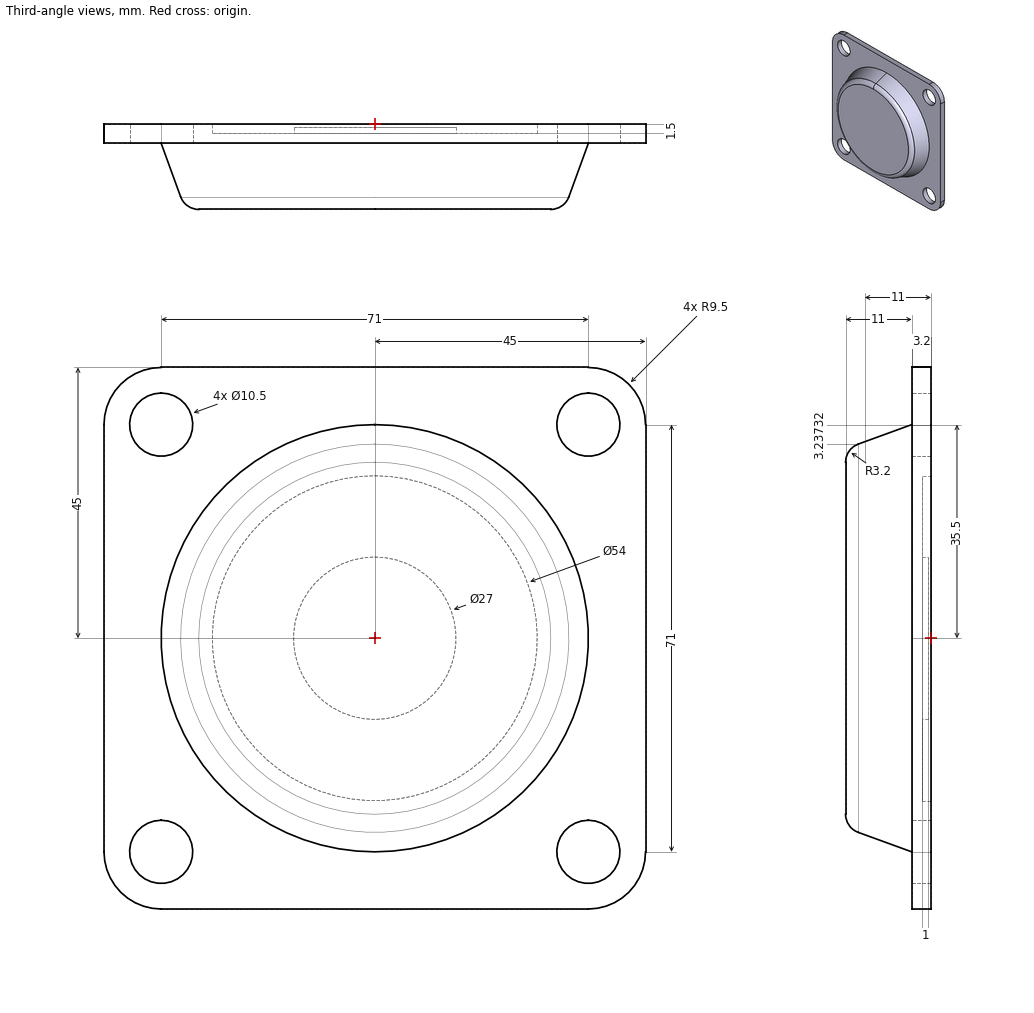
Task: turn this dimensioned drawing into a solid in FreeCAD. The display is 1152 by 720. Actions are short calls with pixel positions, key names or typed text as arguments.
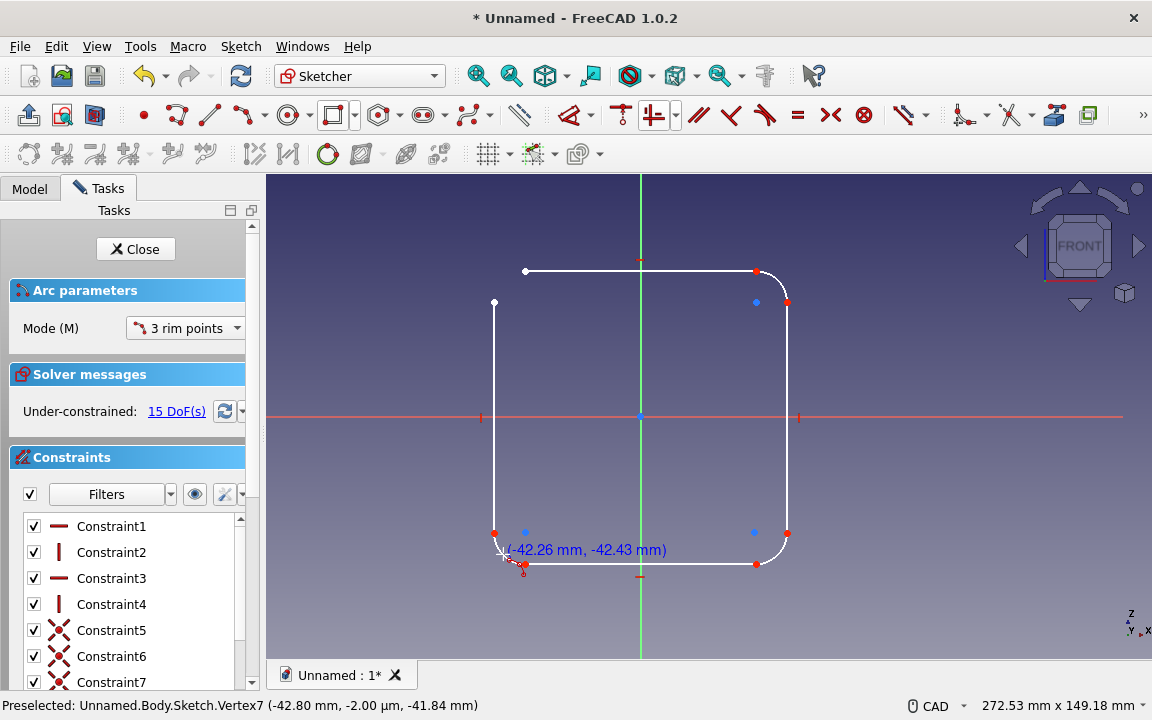
click(494, 302)
click(525, 271)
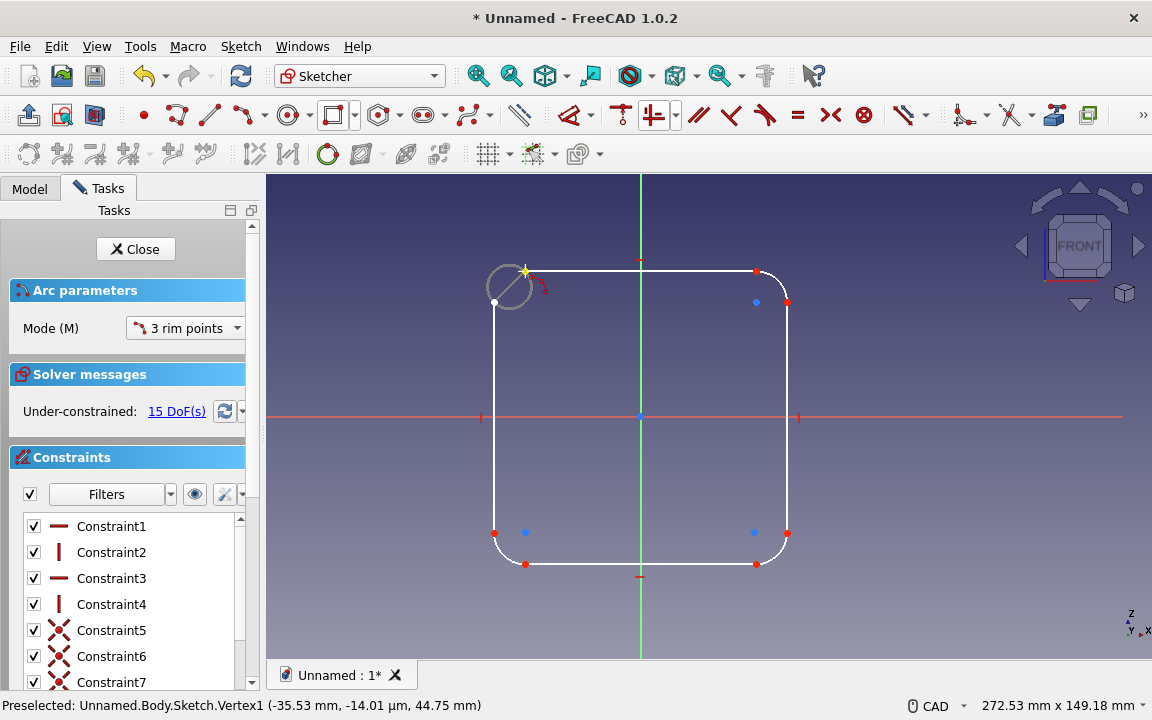
scroll(503, 280, up, 3)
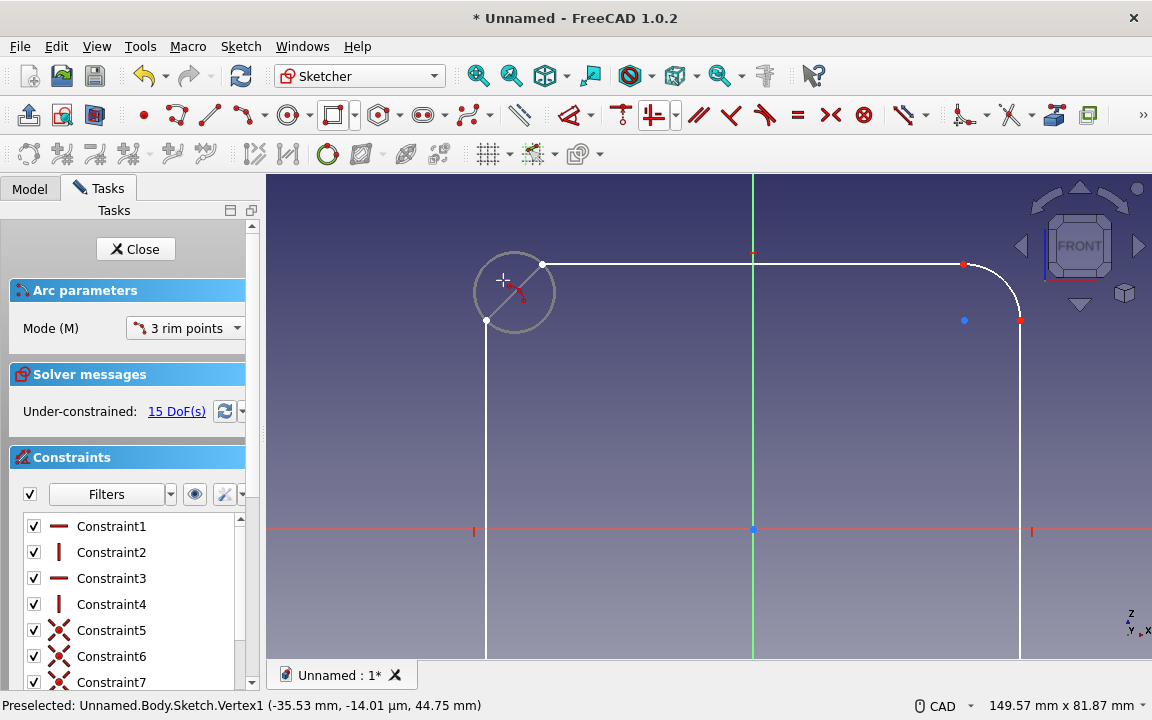
click(503, 279)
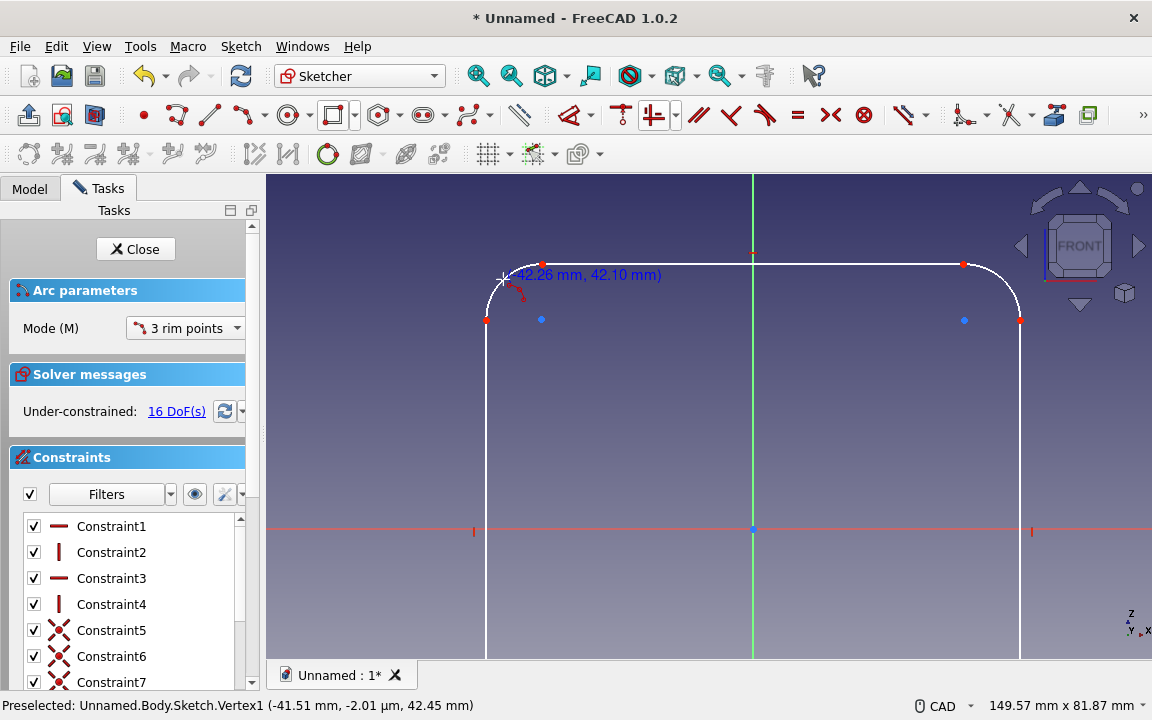
key(g)
key(c)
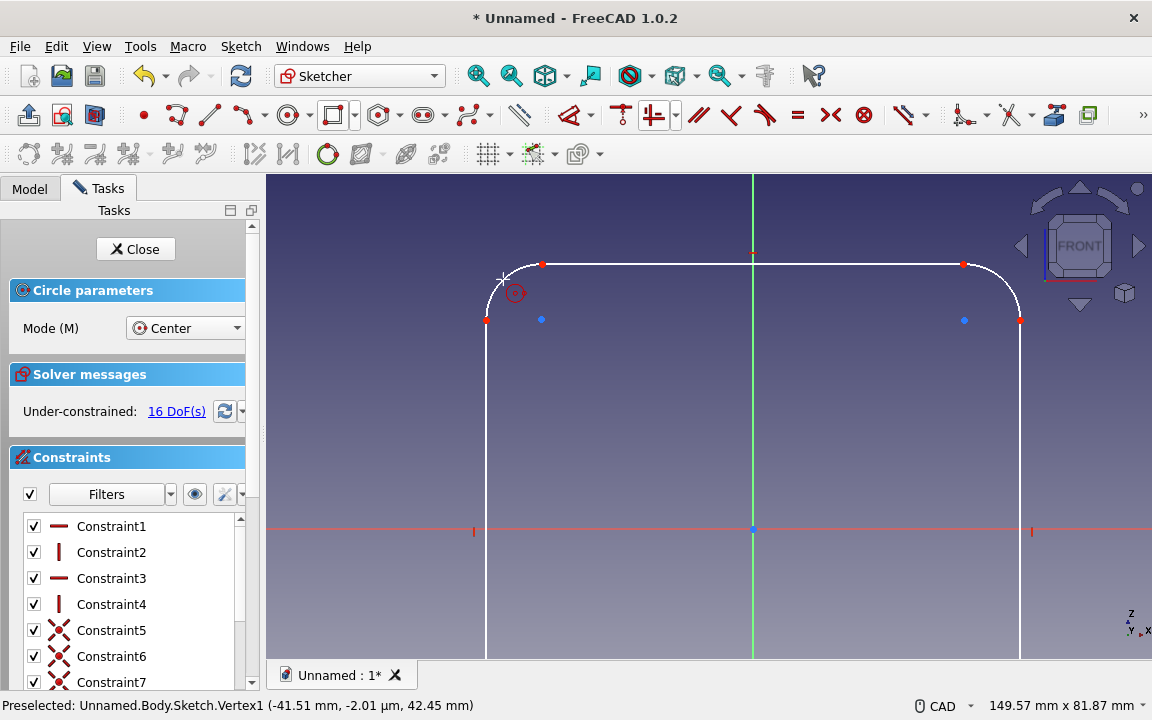
click(543, 319)
move(565, 297)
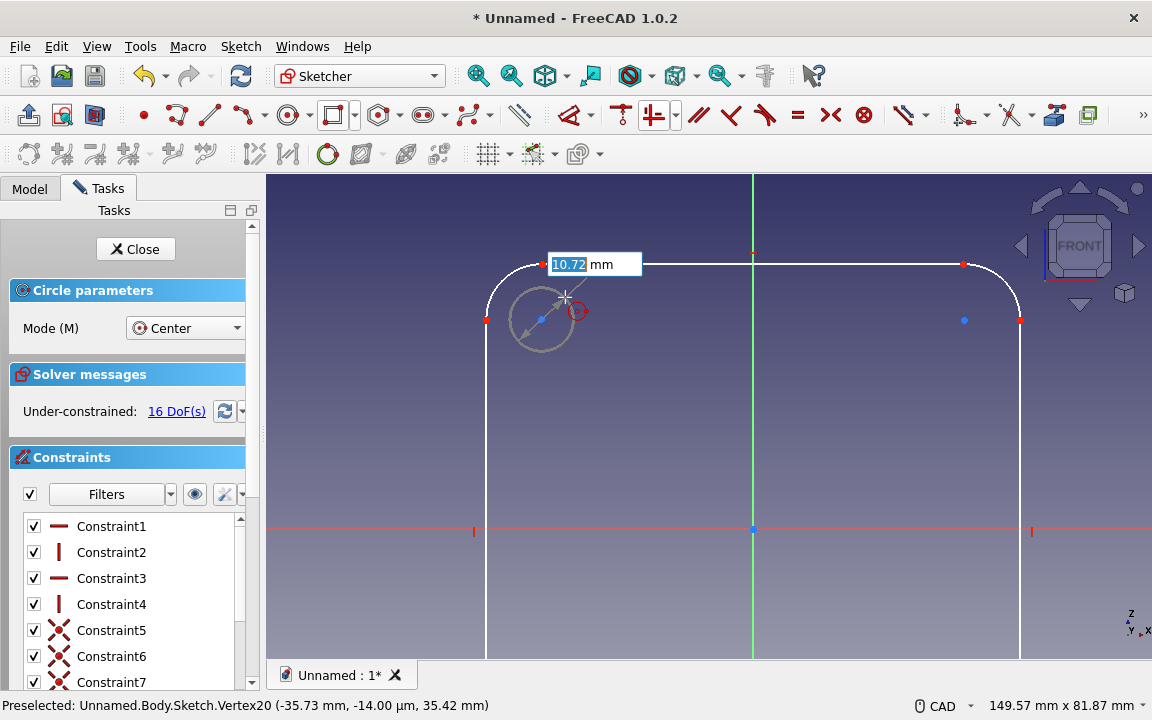
text(10.5)
key(Return)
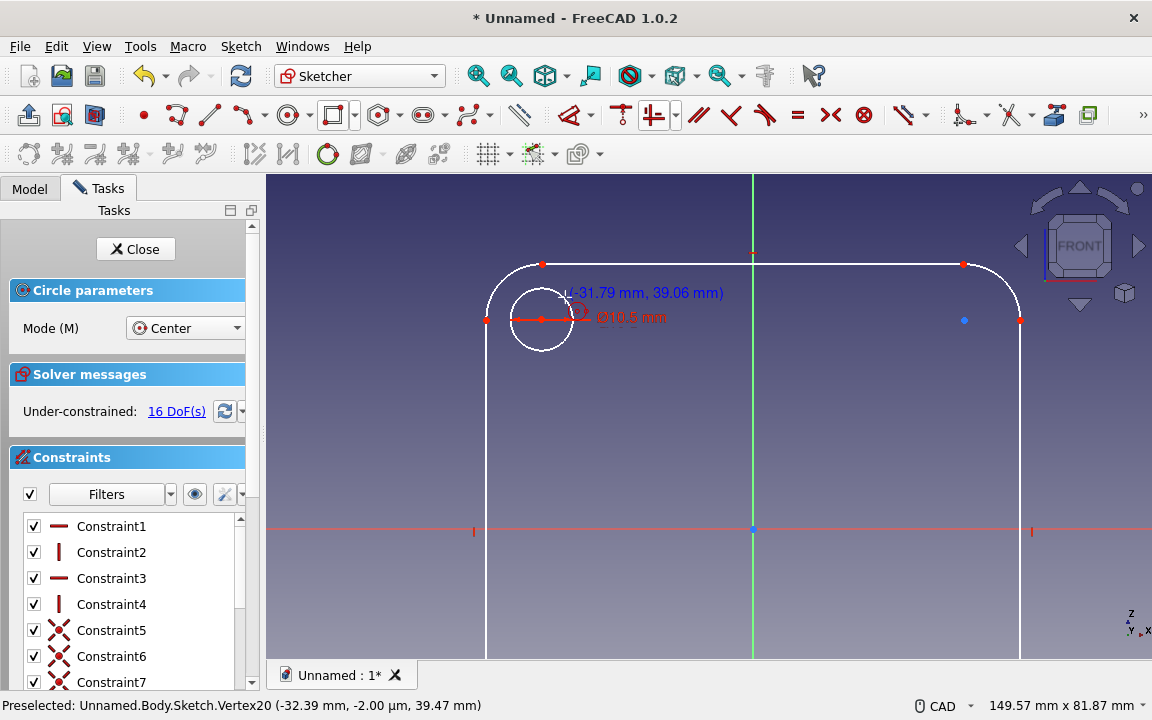
click(964, 319)
move(986, 297)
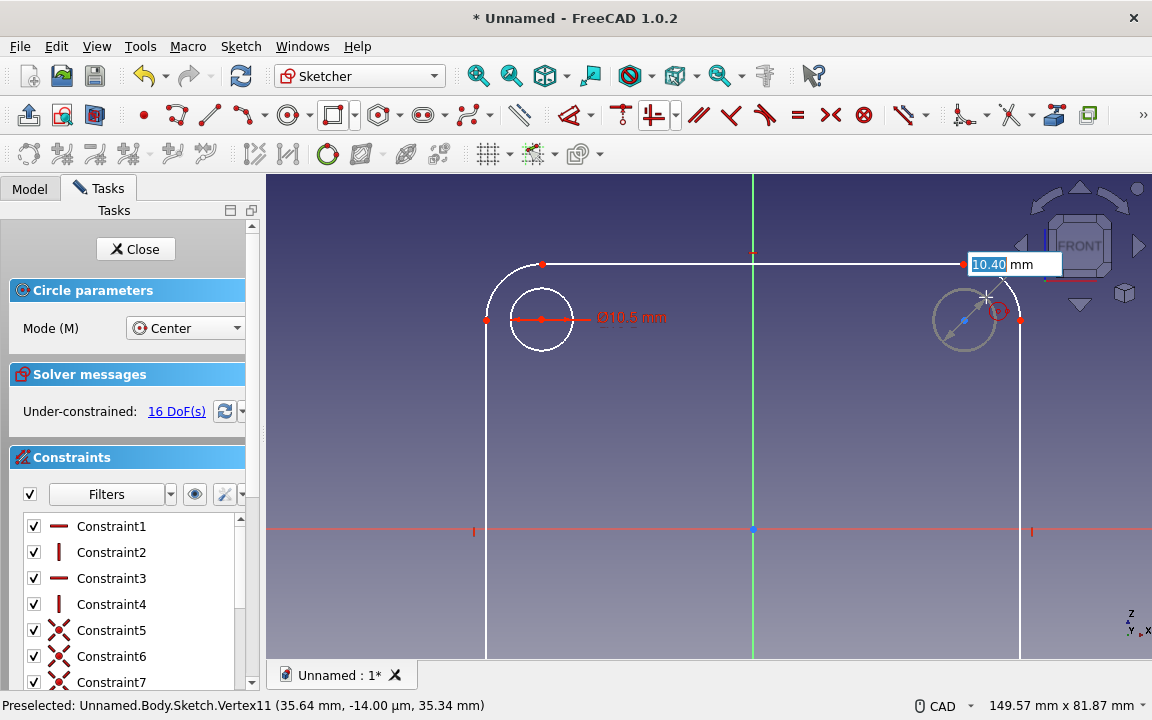
text(10.5)
key(Return)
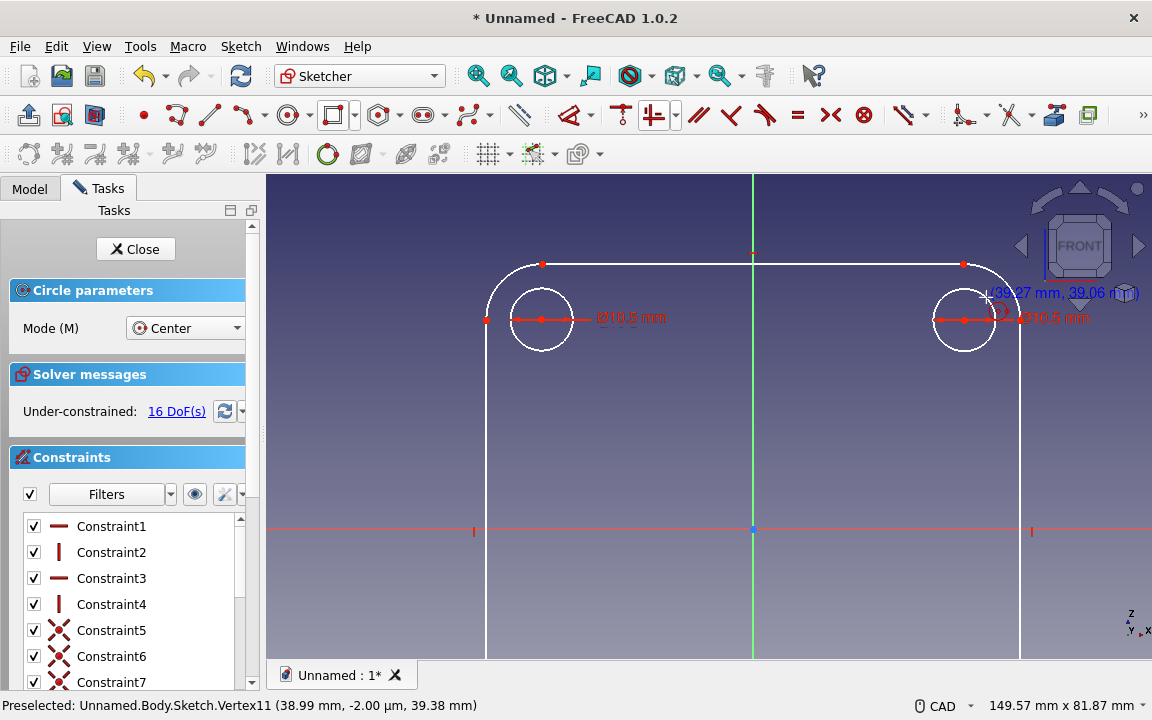
scroll(503, 279, down, 3)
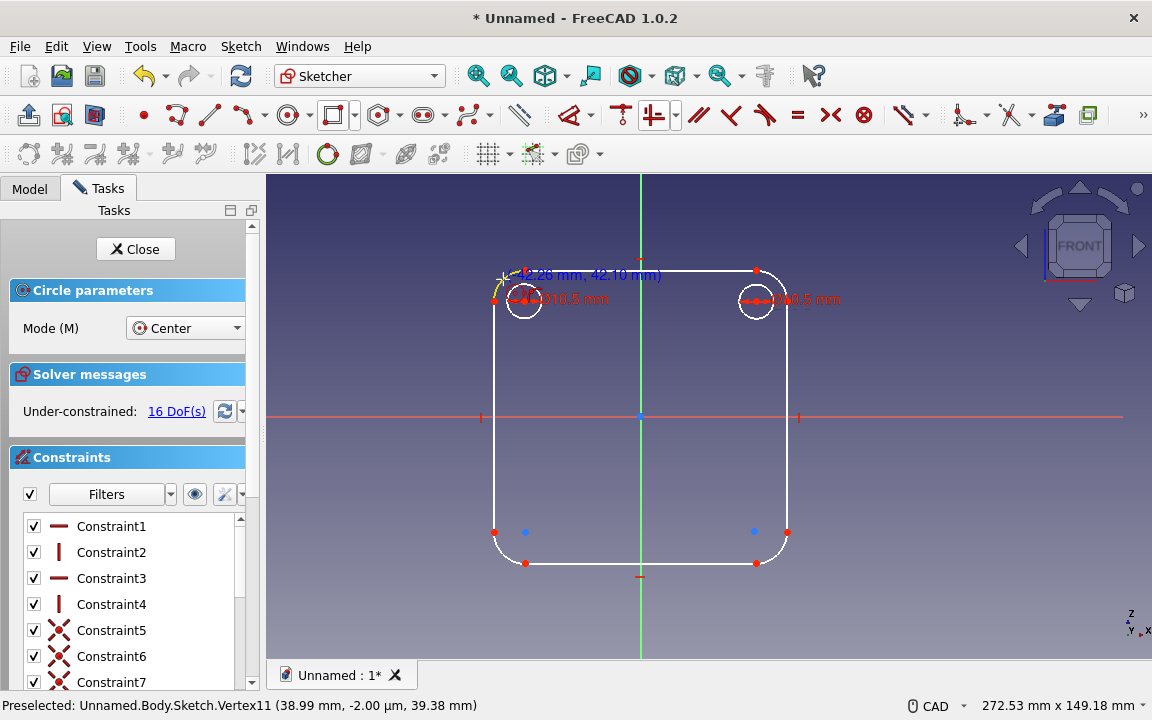
scroll(525, 532, up, 2)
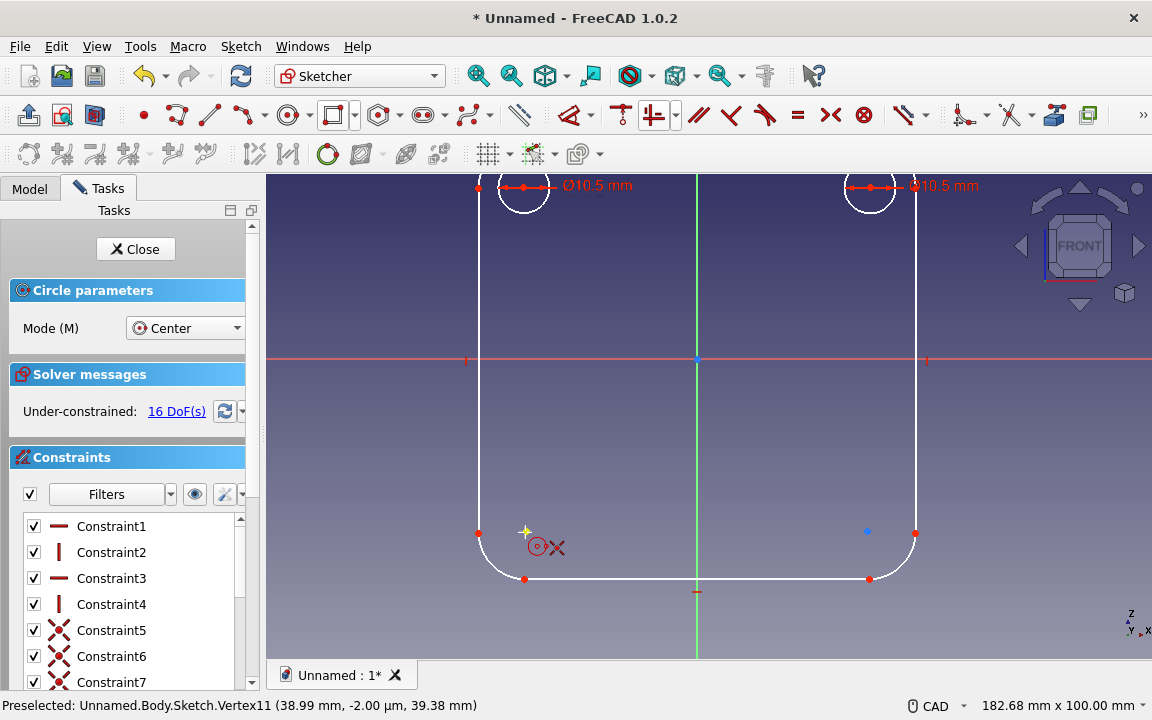
click(525, 532)
move(543, 514)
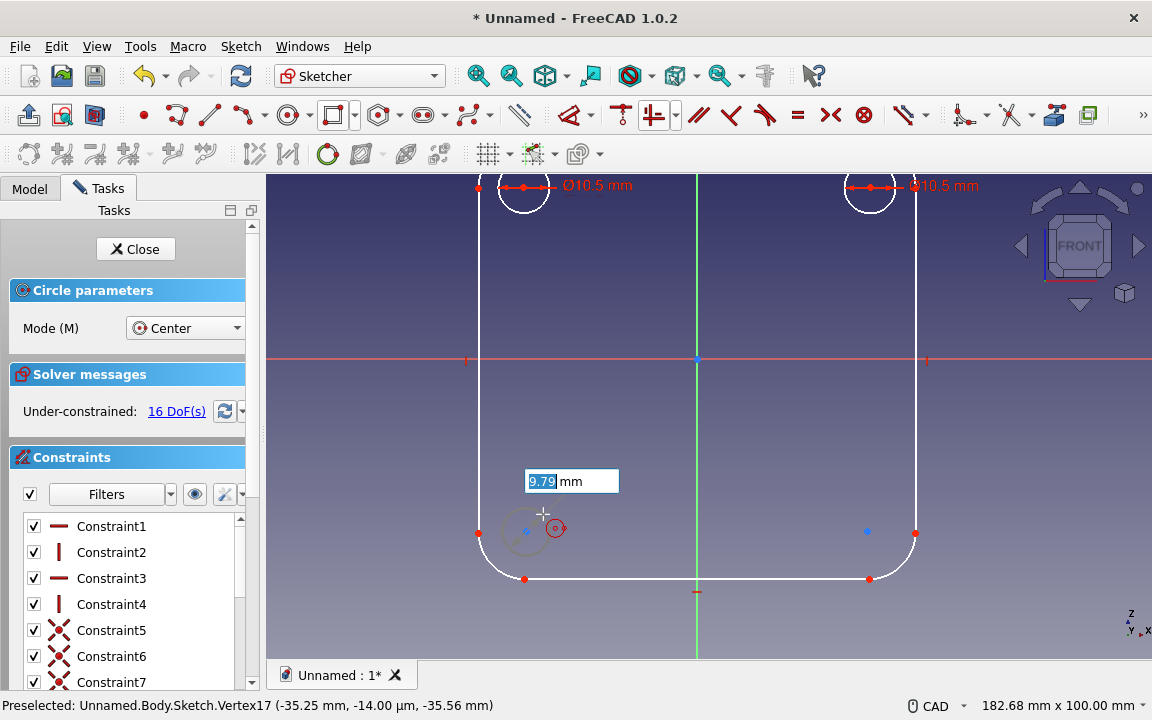
text(10.5)
key(Return)